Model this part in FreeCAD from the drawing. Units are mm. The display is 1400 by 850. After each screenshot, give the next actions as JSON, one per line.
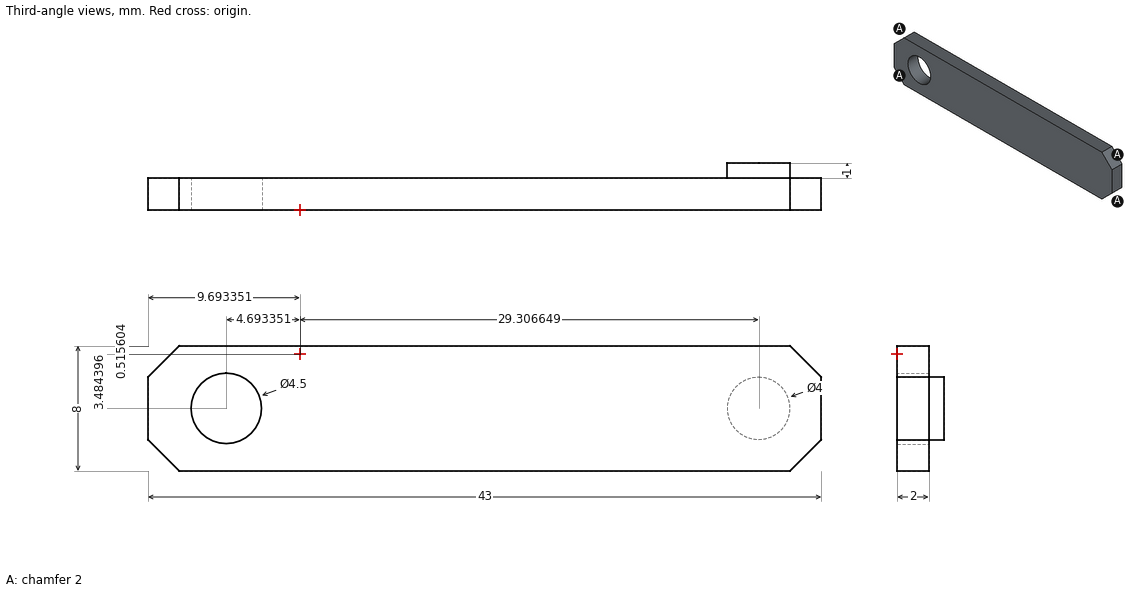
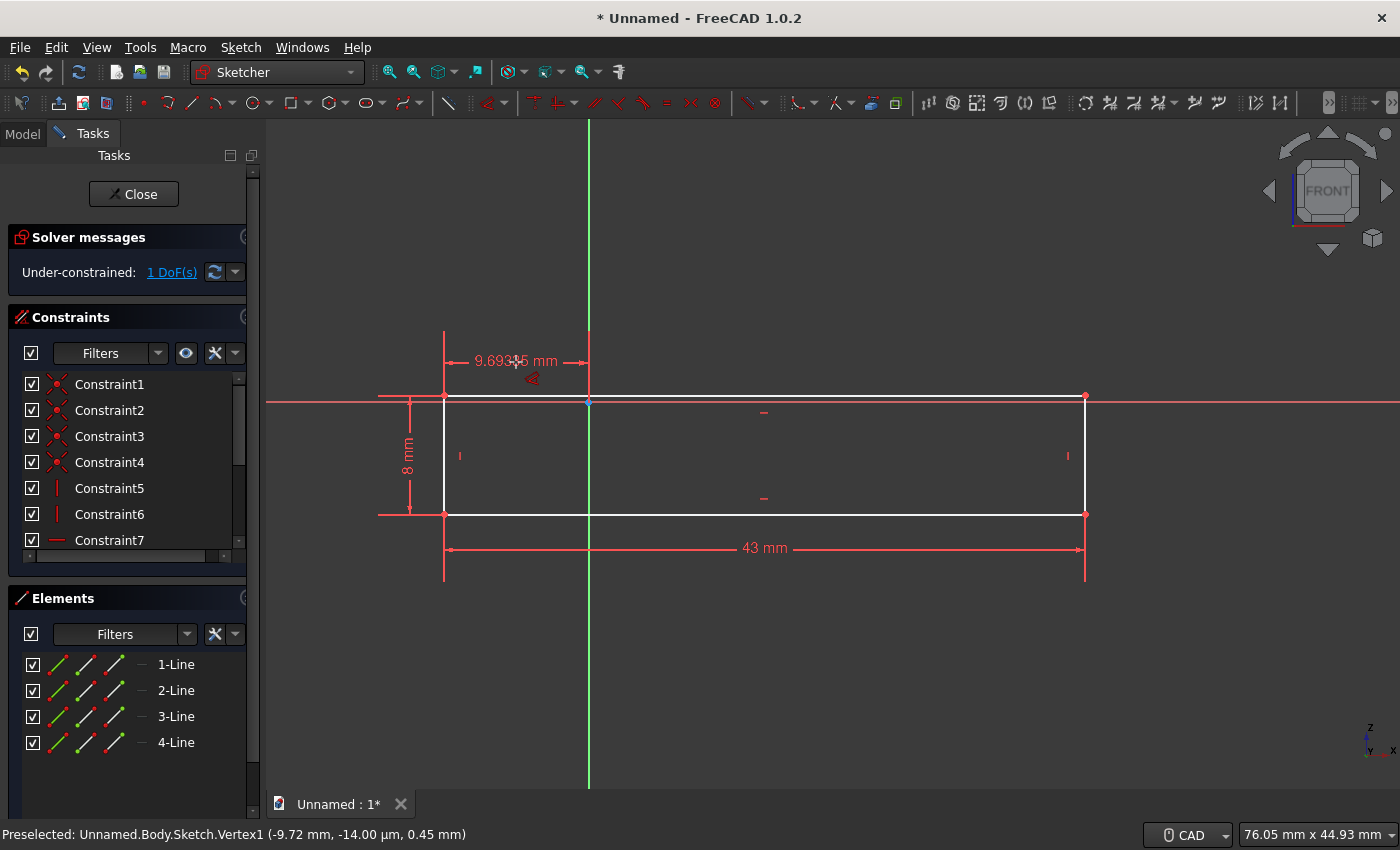
{"action": "scroll", "coordinate": [444, 396], "scroll_direction": "up", "scroll_amount": 9}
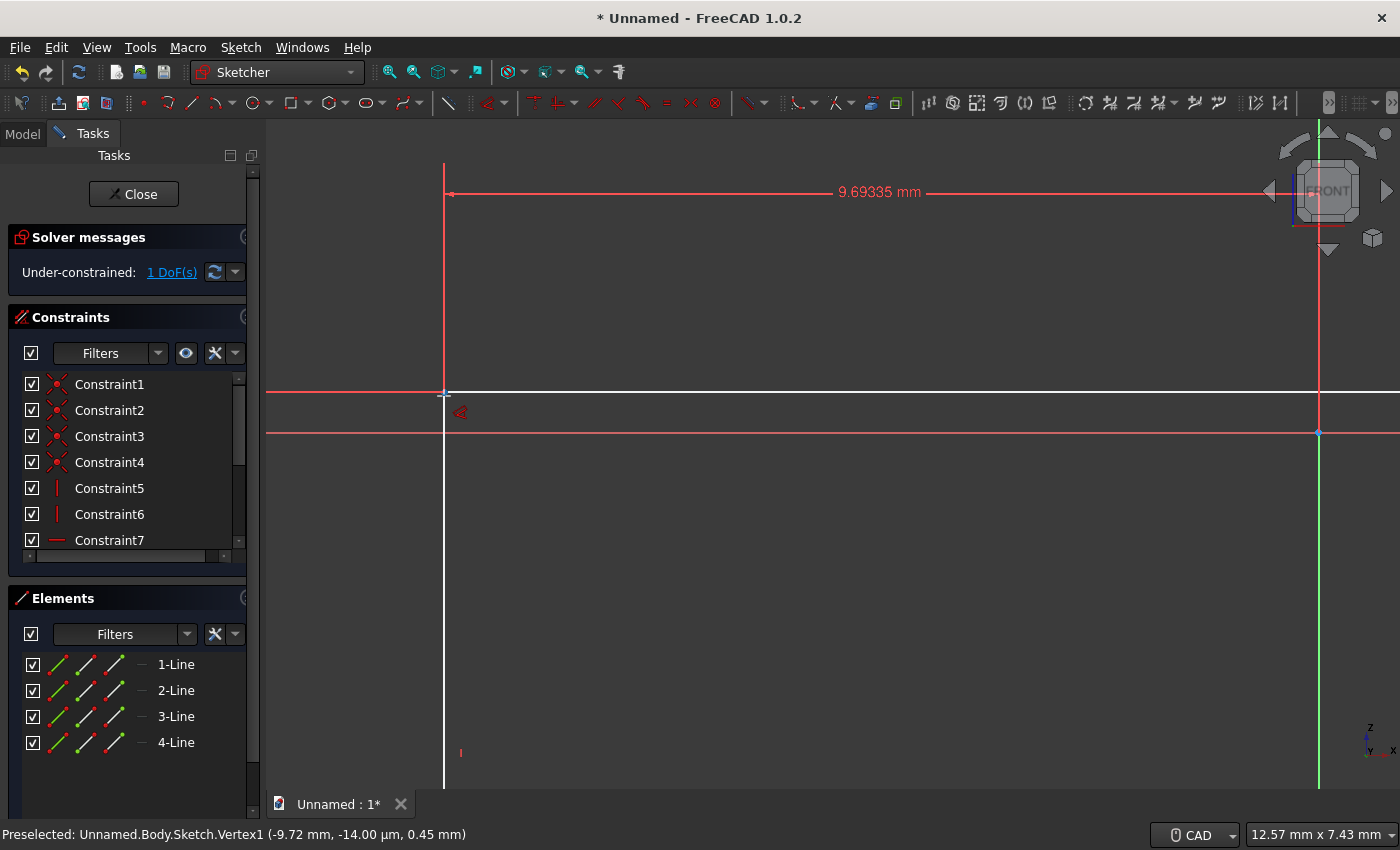
{"action": "left_click", "coordinate": [444, 392]}
{"action": "left_click", "coordinate": [410, 412]}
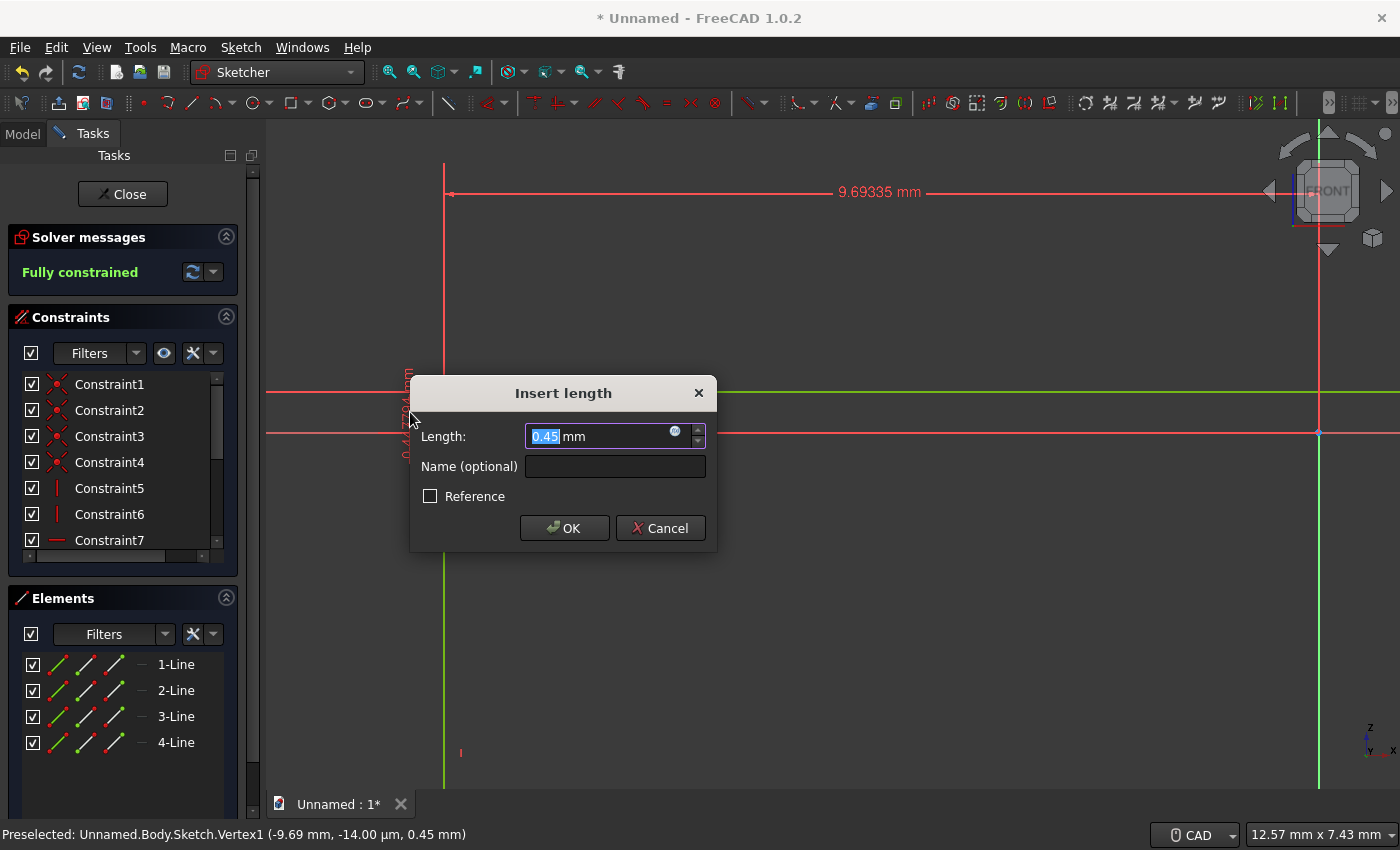
{"action": "type", "text": "0.515604"}
{"action": "key", "text": "Return"}
{"action": "key", "text": "Escape"}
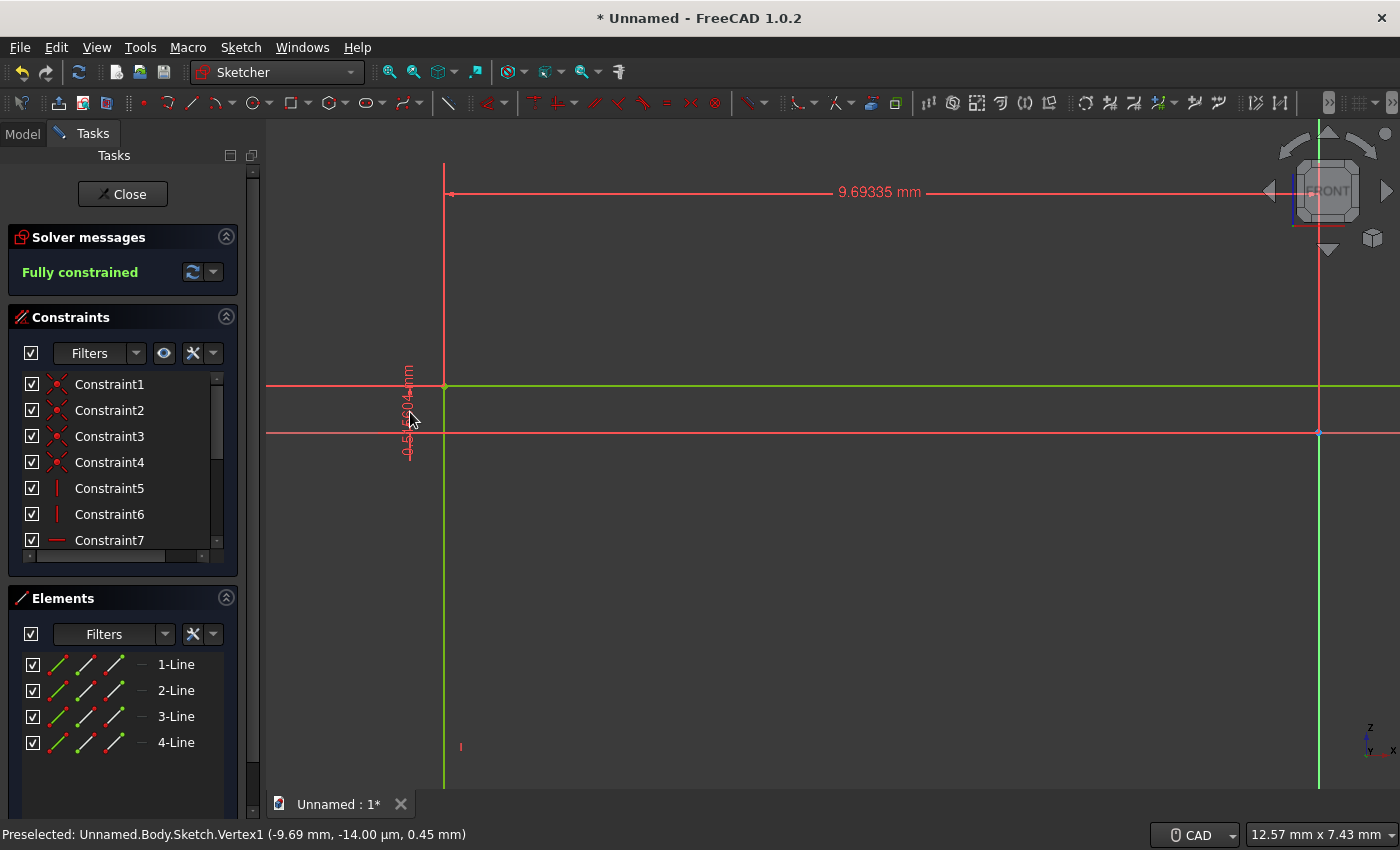
{"action": "left_click", "coordinate": [123, 194]}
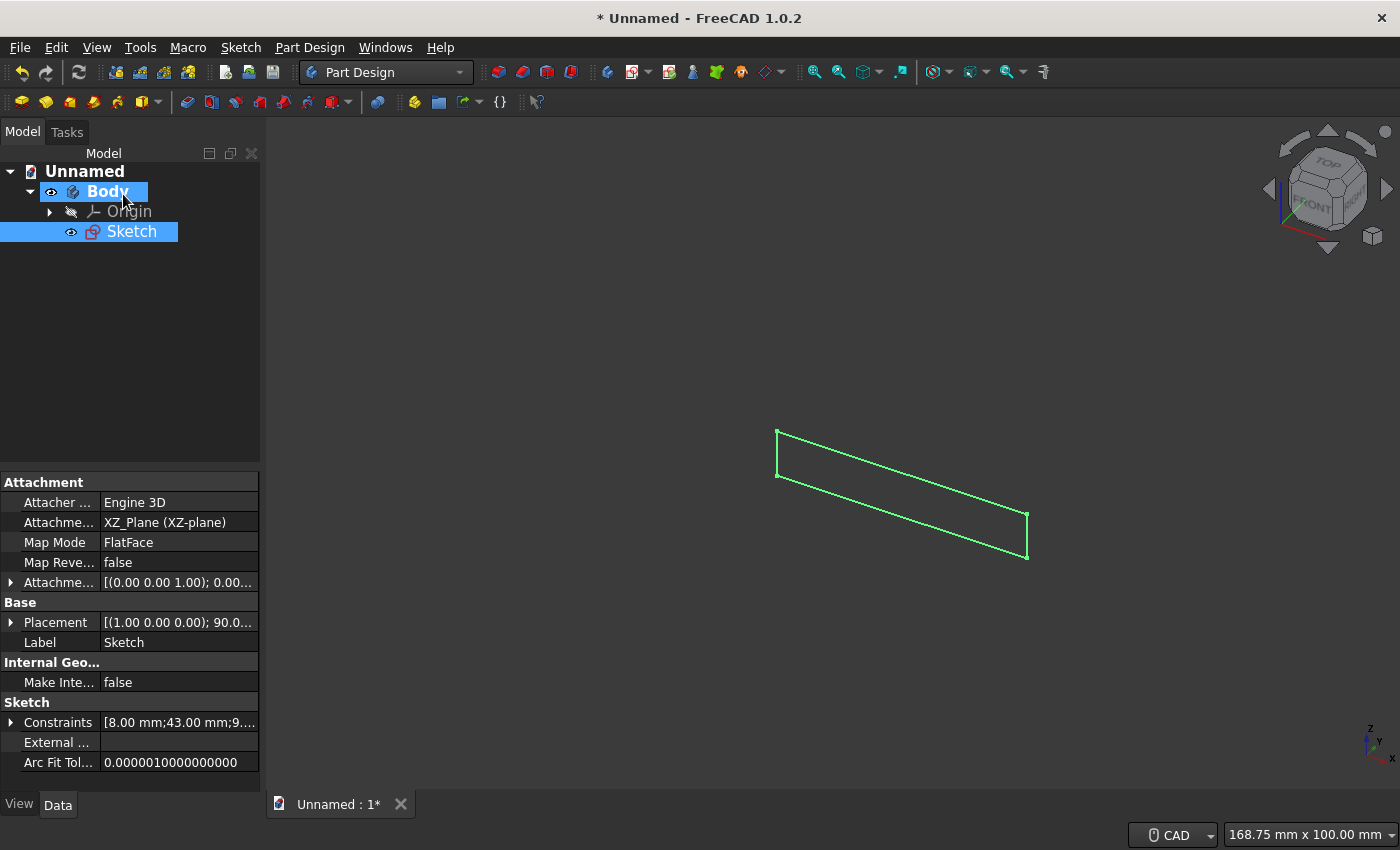
{"action": "left_click", "coordinate": [22, 102]}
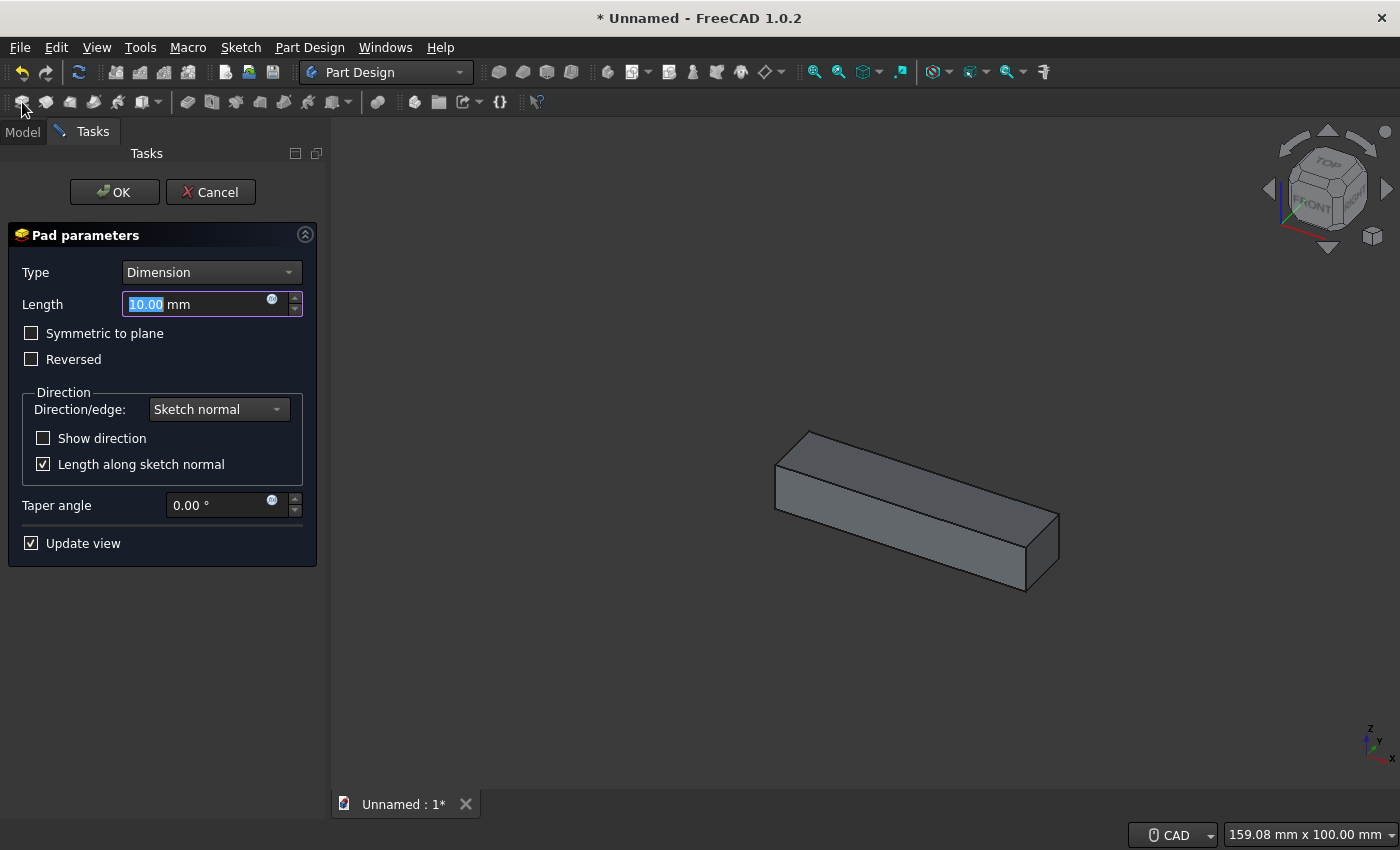
{"action": "type", "text": "2"}
{"action": "key", "text": "Tab"}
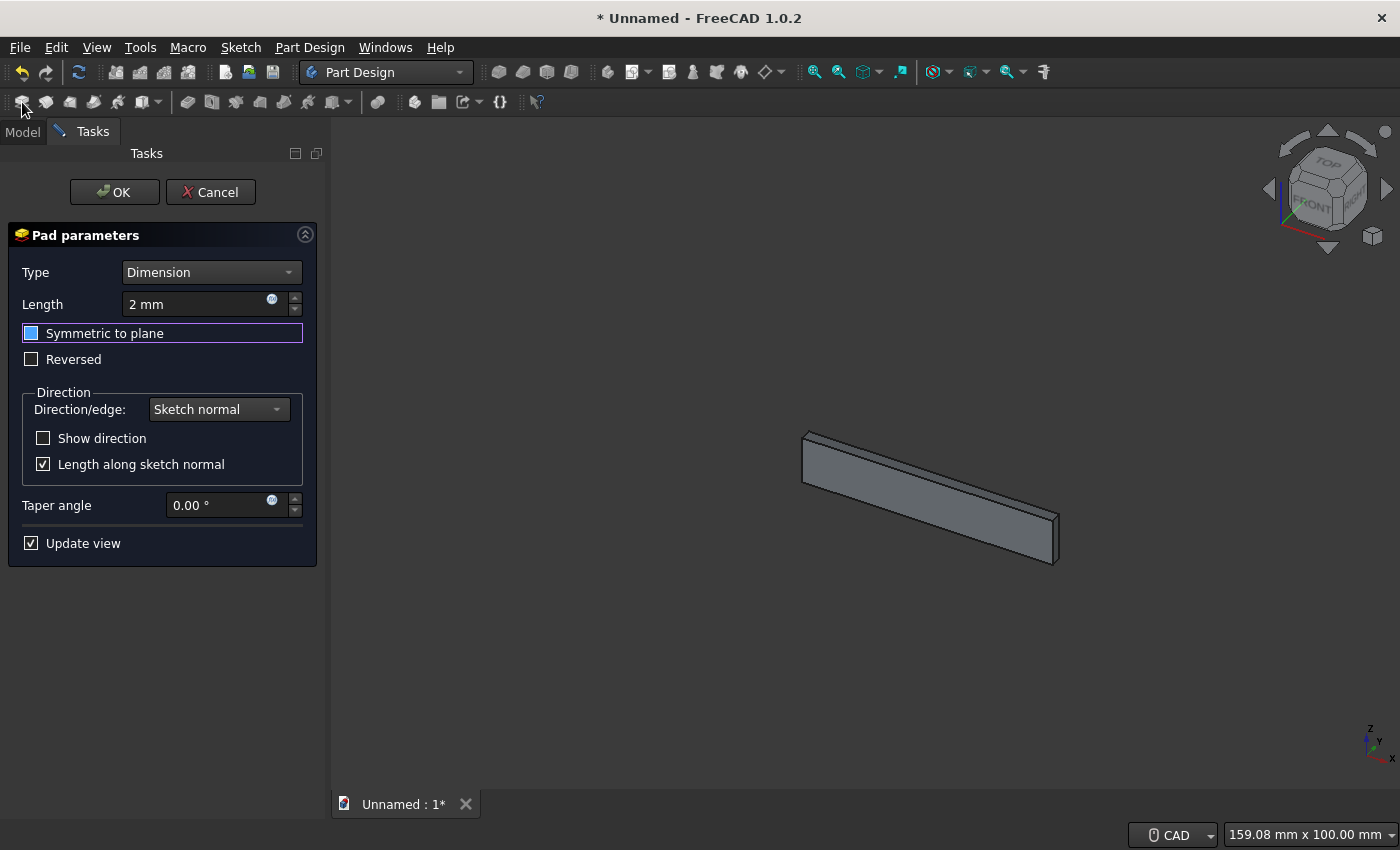
{"action": "left_click", "coordinate": [30, 359]}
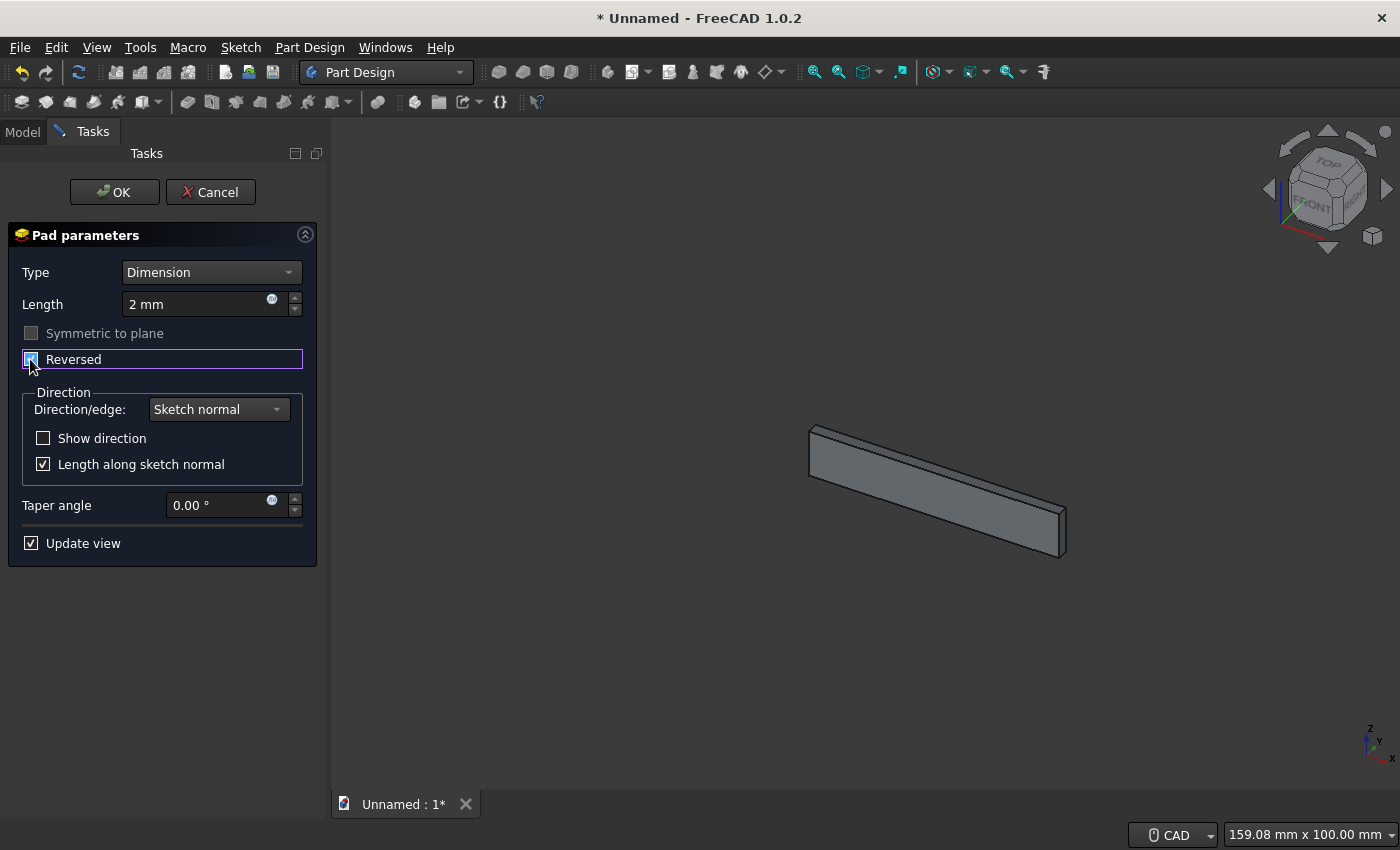
{"action": "left_click", "coordinate": [115, 192]}